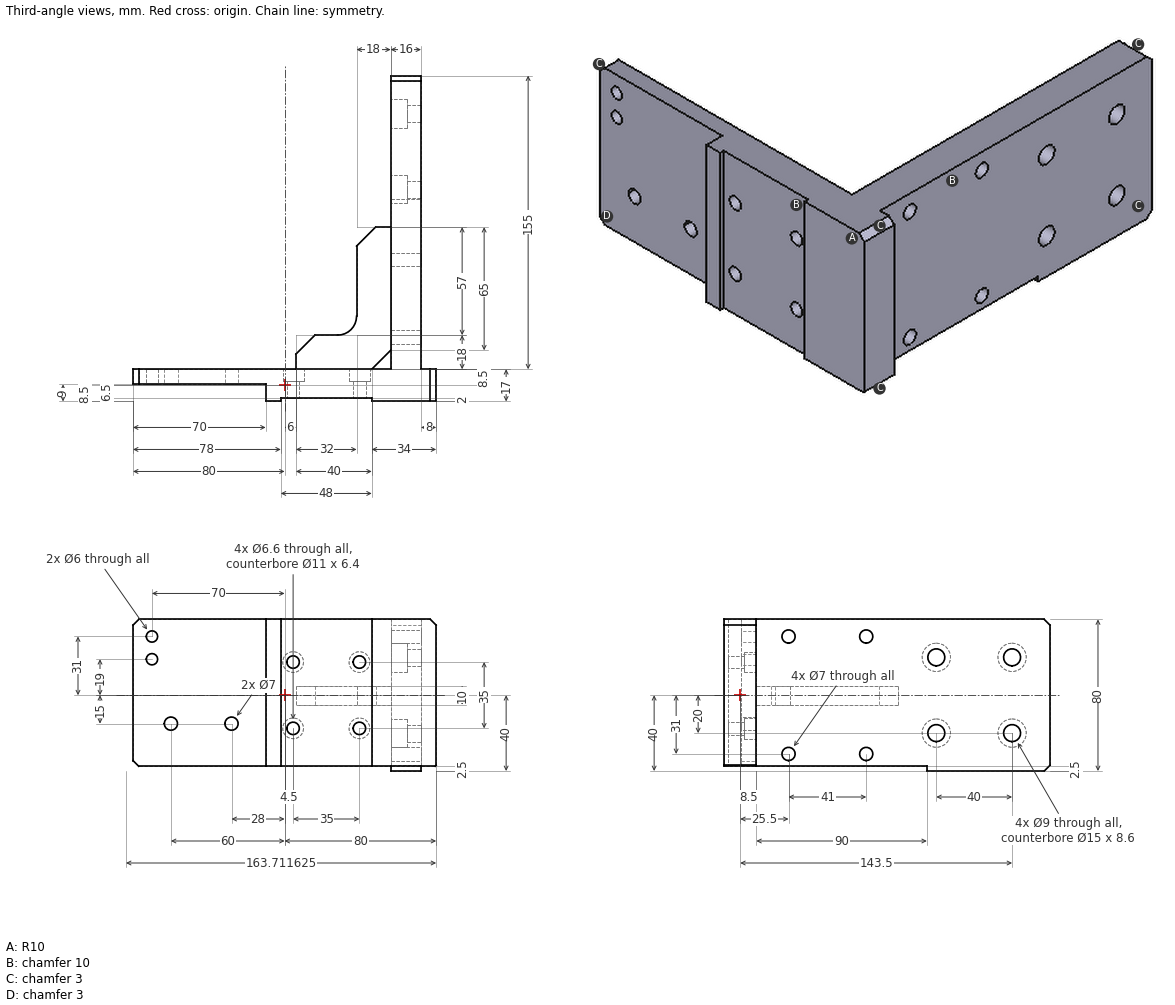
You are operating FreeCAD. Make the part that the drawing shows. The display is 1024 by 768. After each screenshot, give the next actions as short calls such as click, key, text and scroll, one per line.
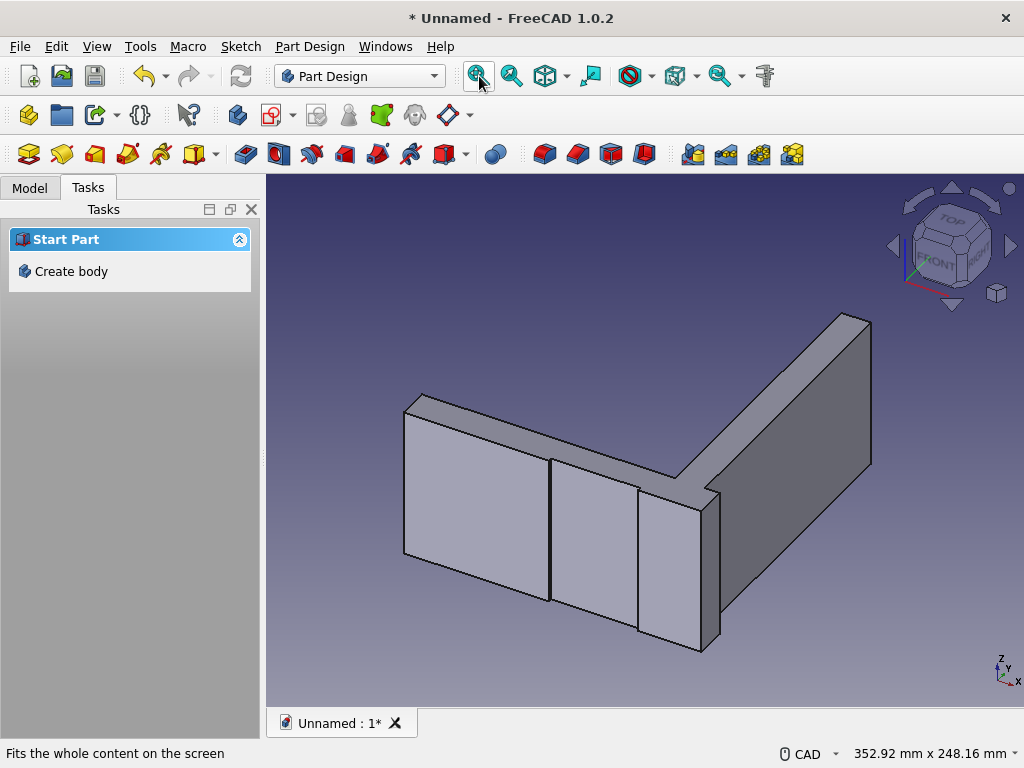
key(6)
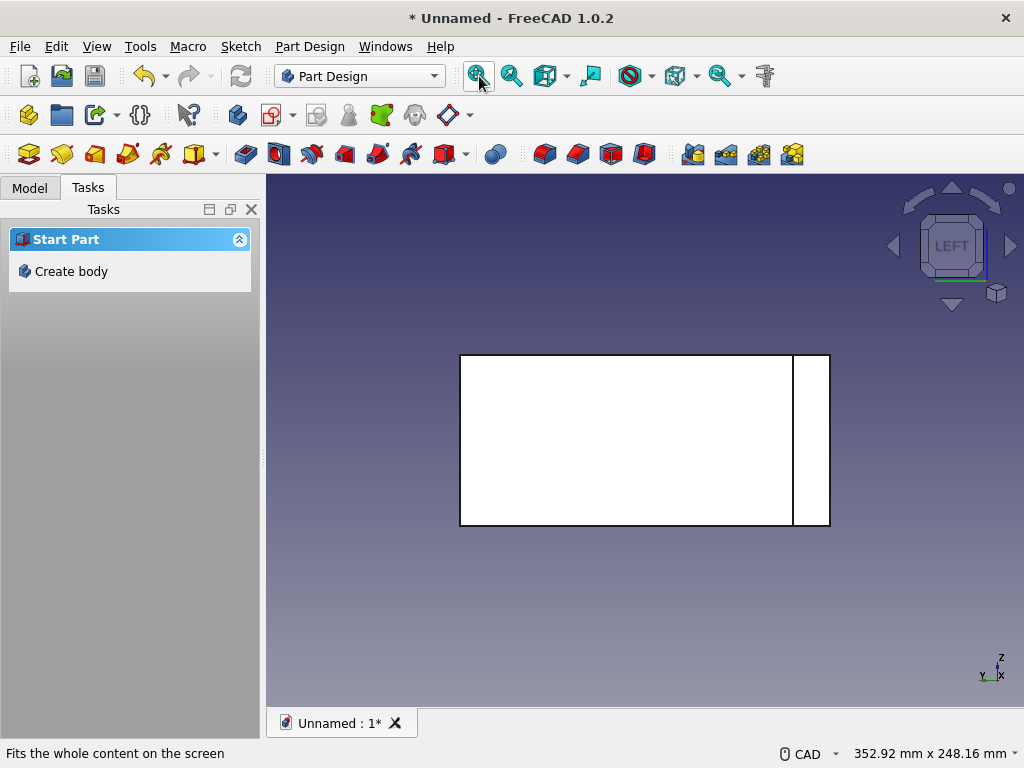
click(579, 439)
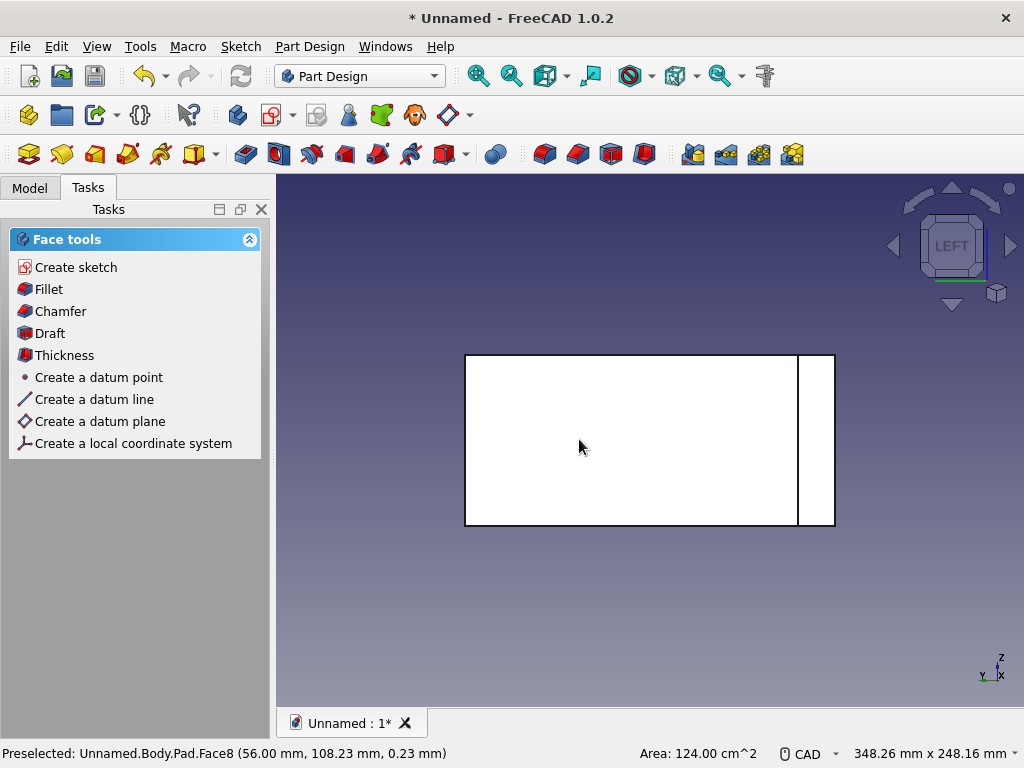
click(270, 116)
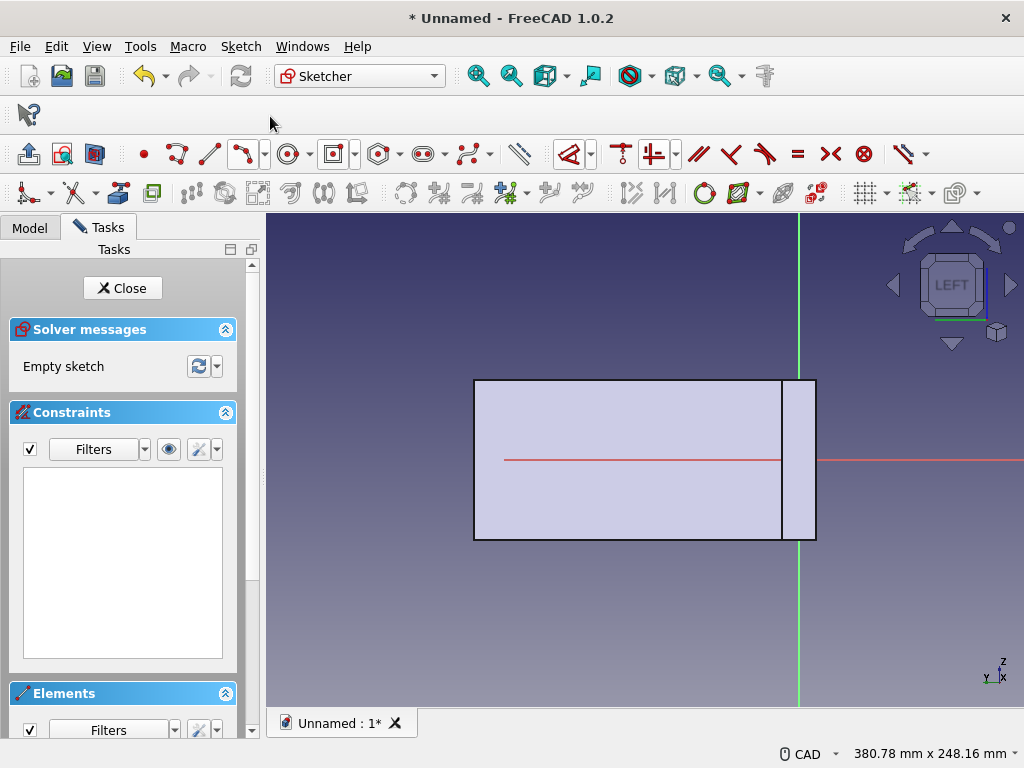
key(q)
key(s)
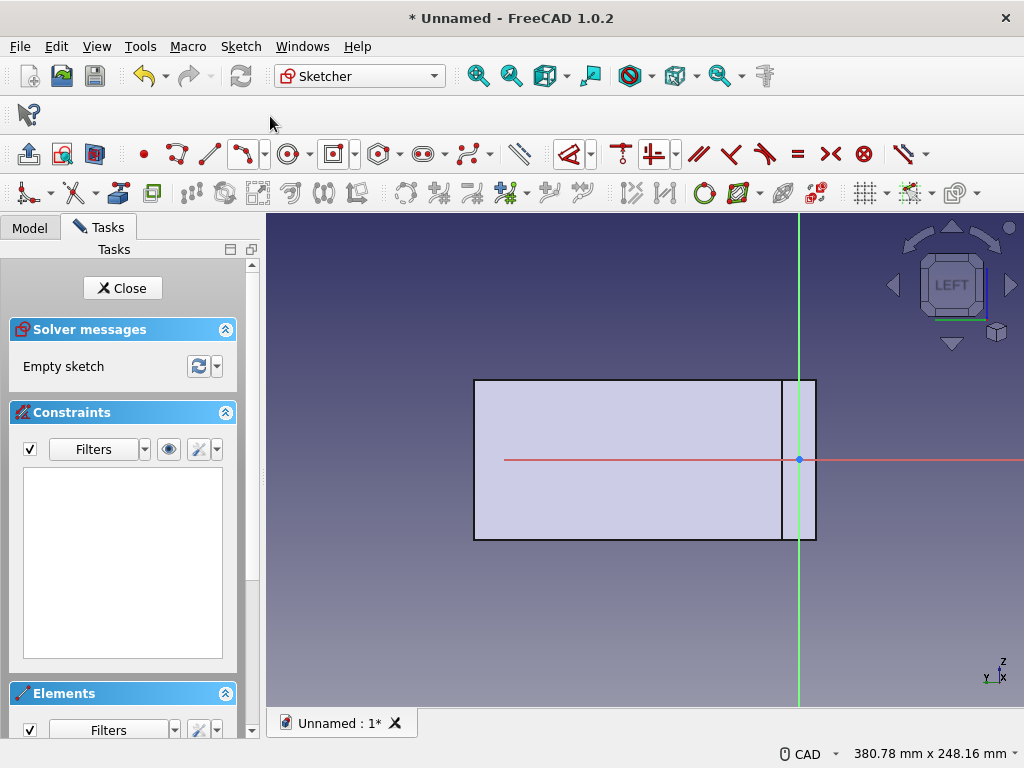
scroll(803, 532, up, 4)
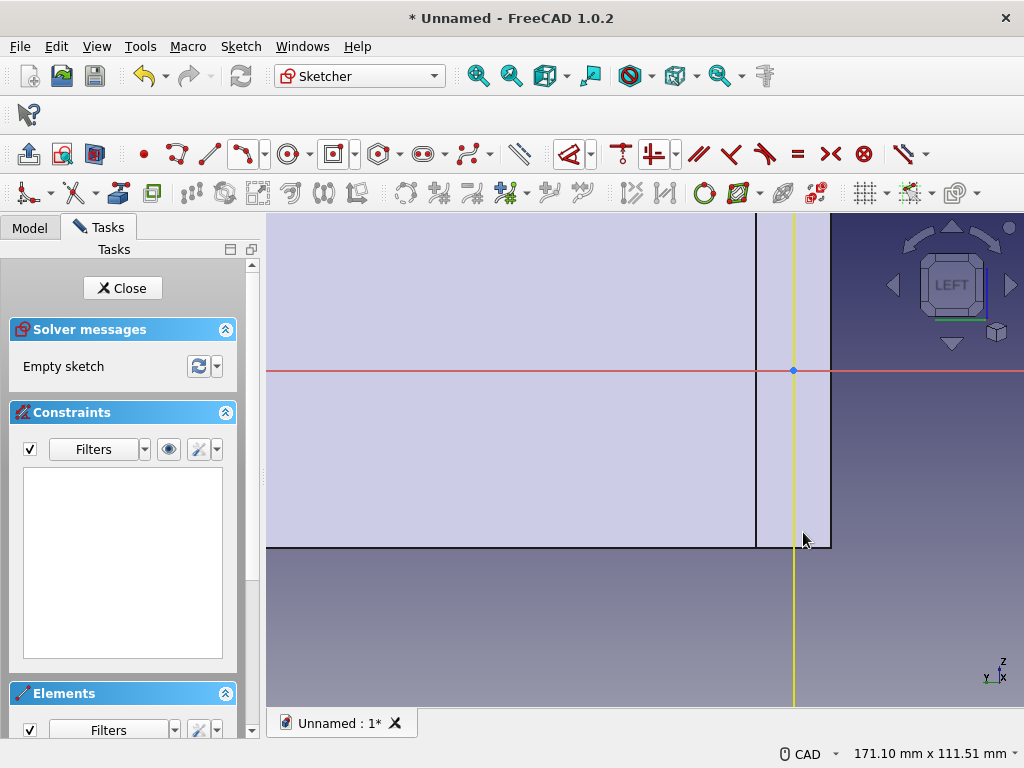
click(354, 154)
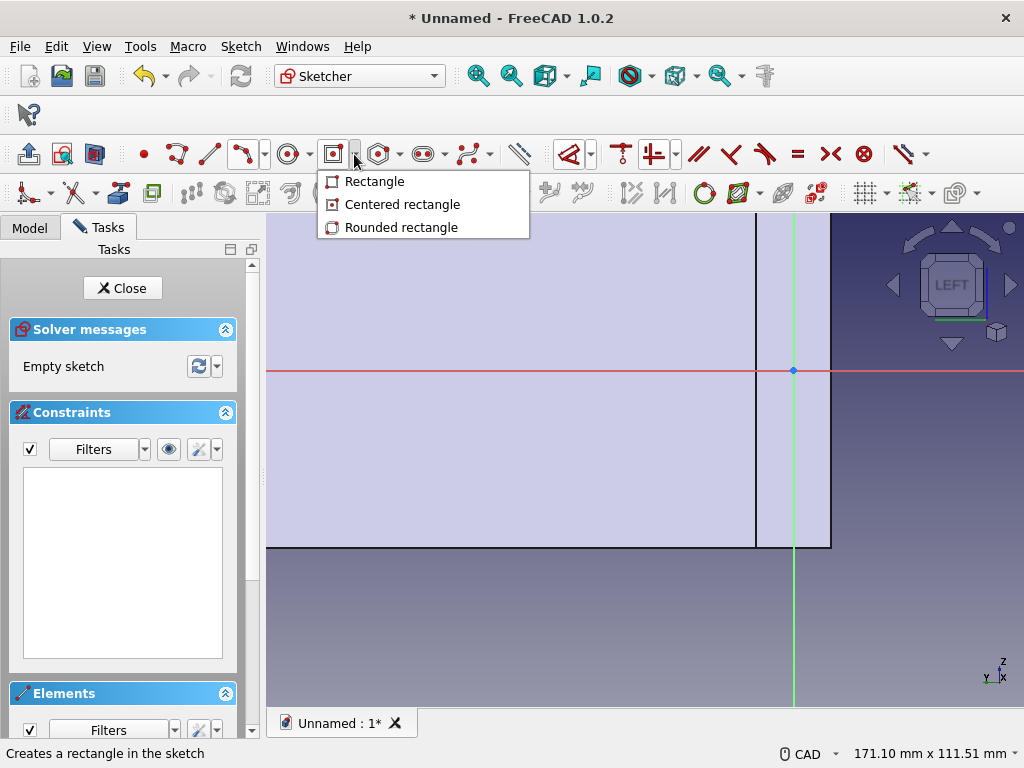
click(424, 182)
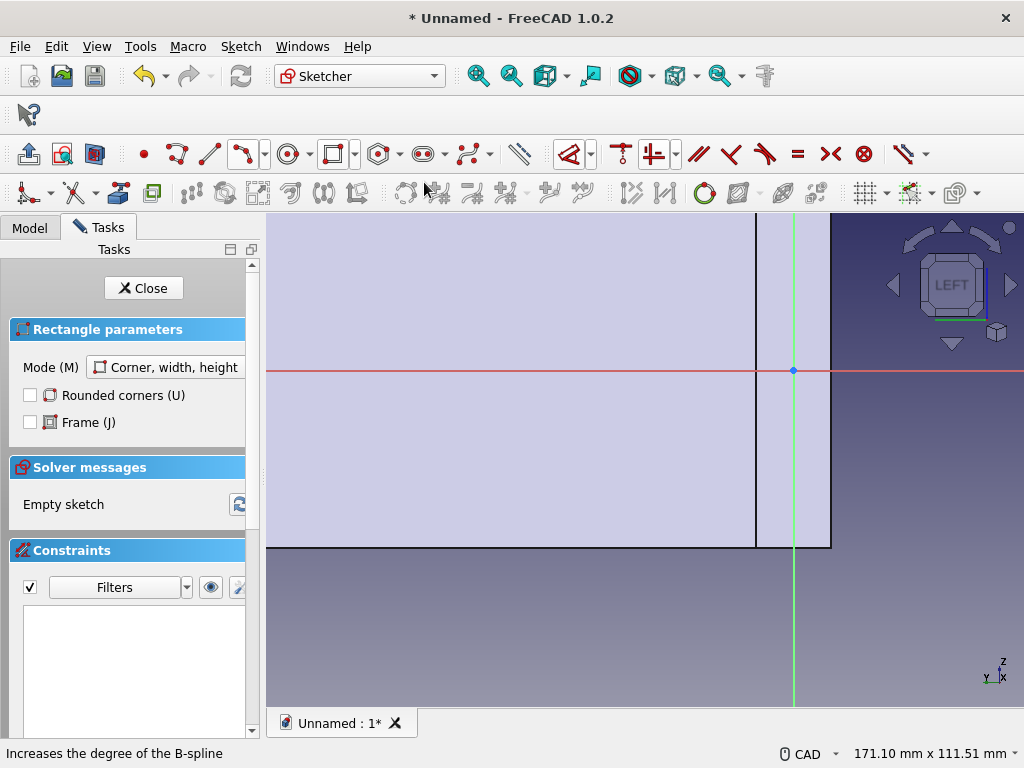
scroll(357, 537, up, 2)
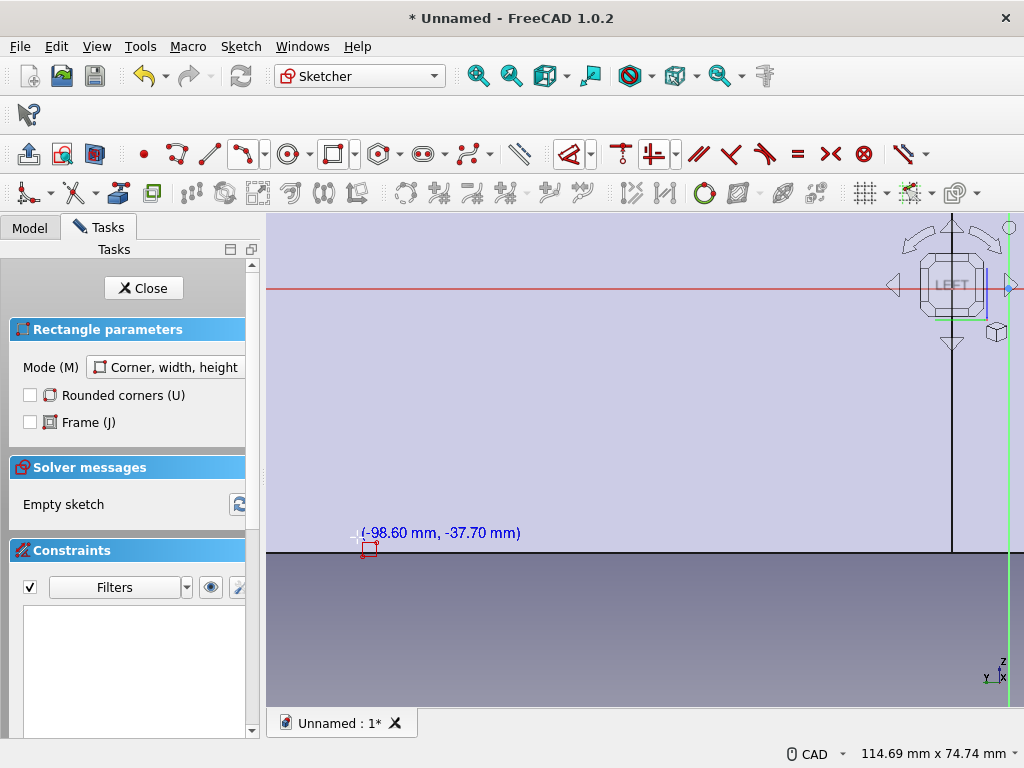
click(358, 537)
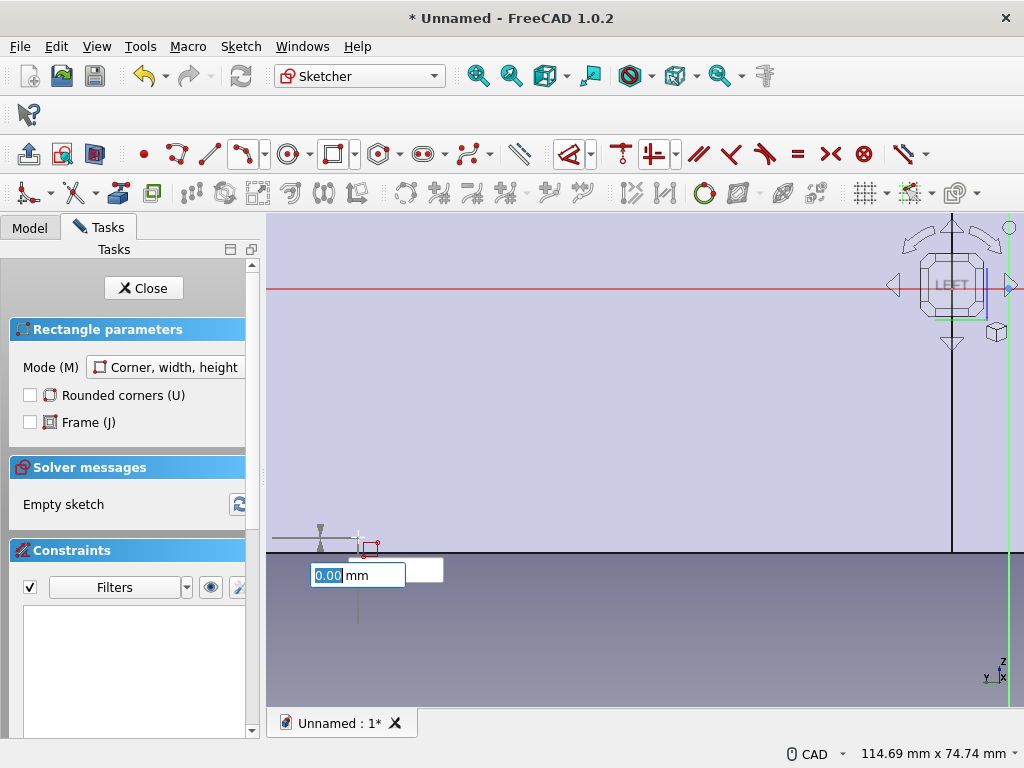
scroll(360, 539, down, 2)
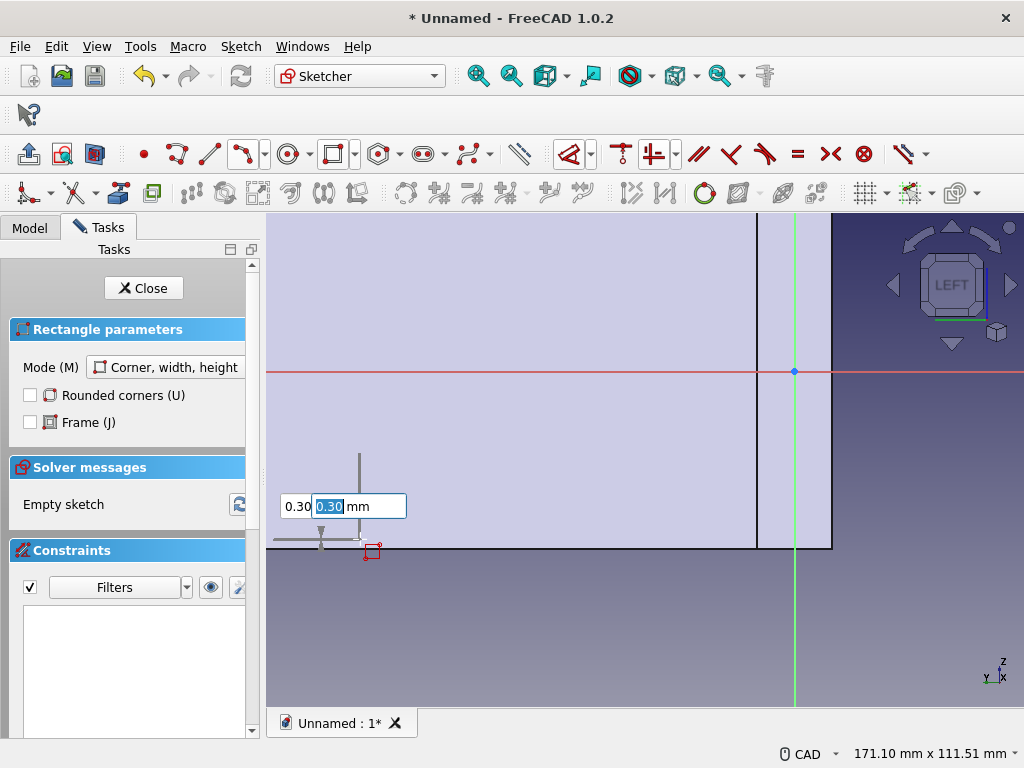
click(757, 549)
key(Escape)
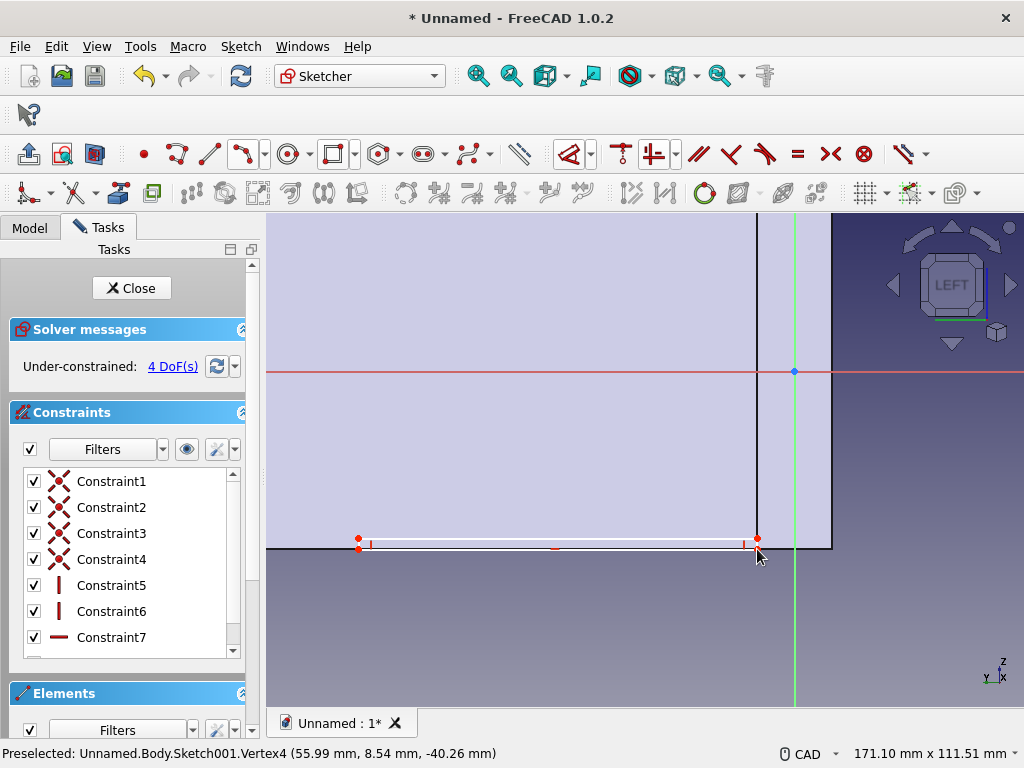
click(478, 550)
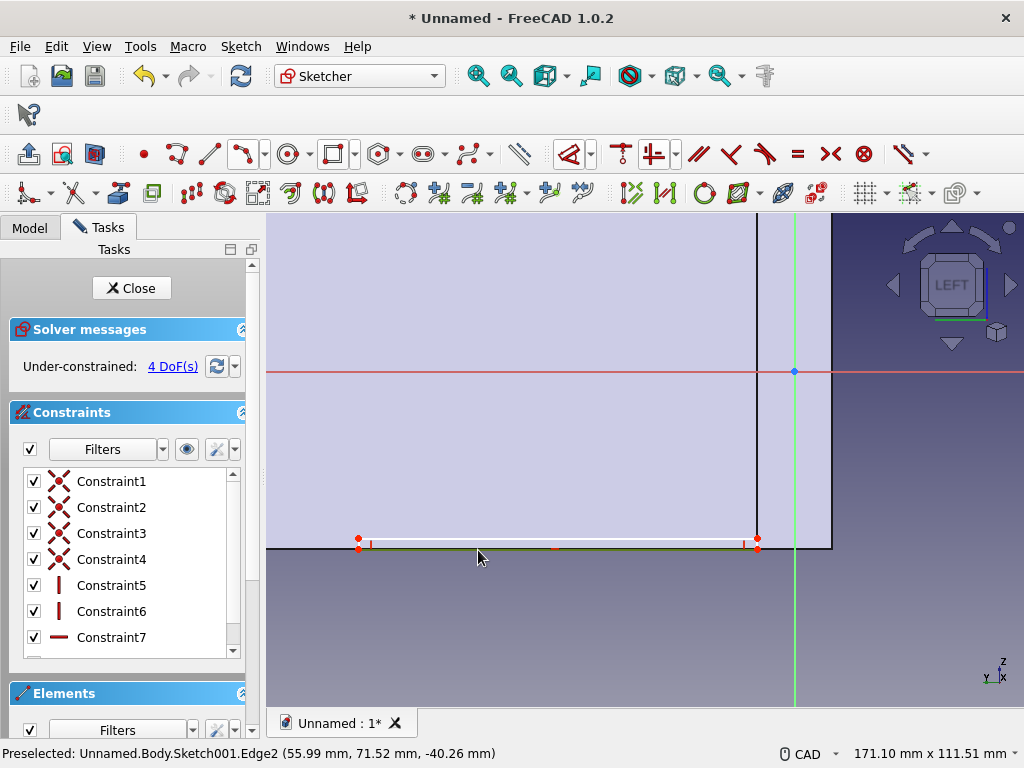
key(l)